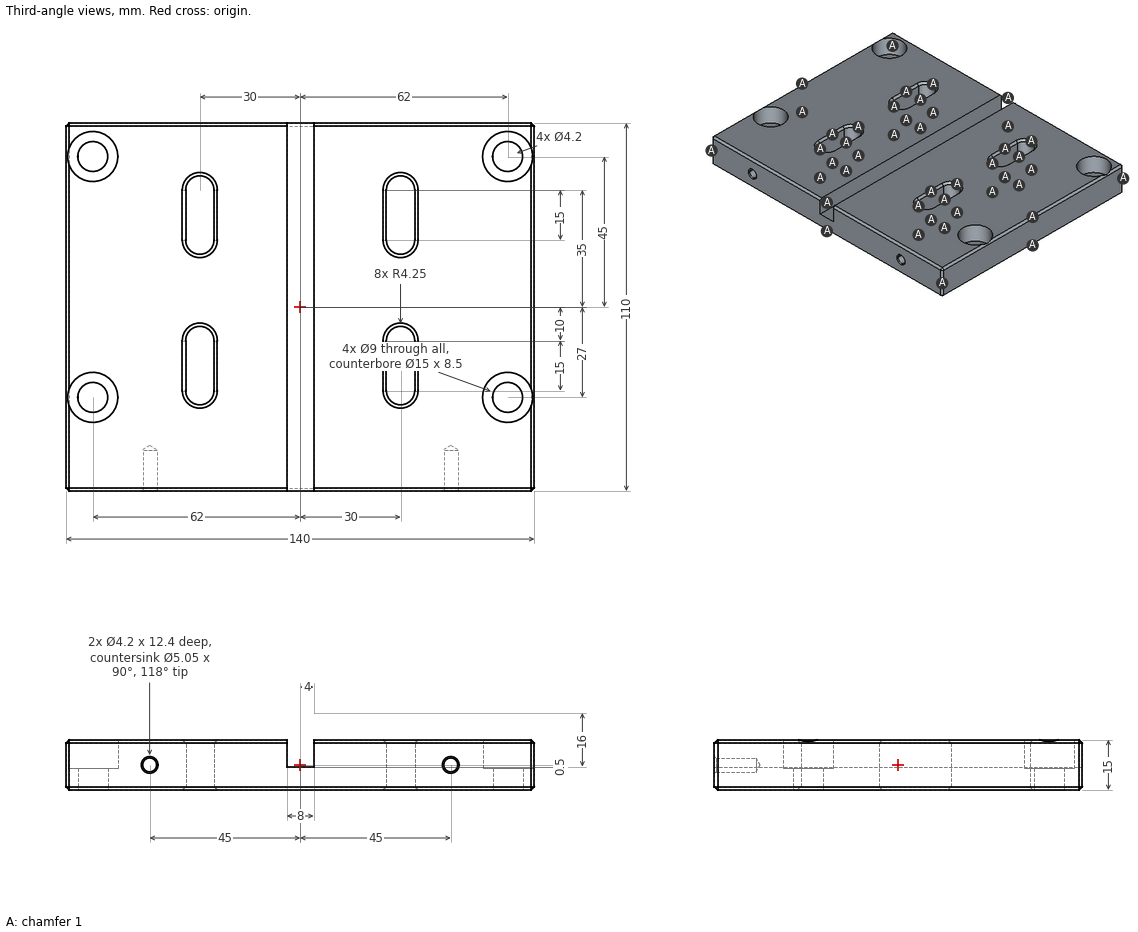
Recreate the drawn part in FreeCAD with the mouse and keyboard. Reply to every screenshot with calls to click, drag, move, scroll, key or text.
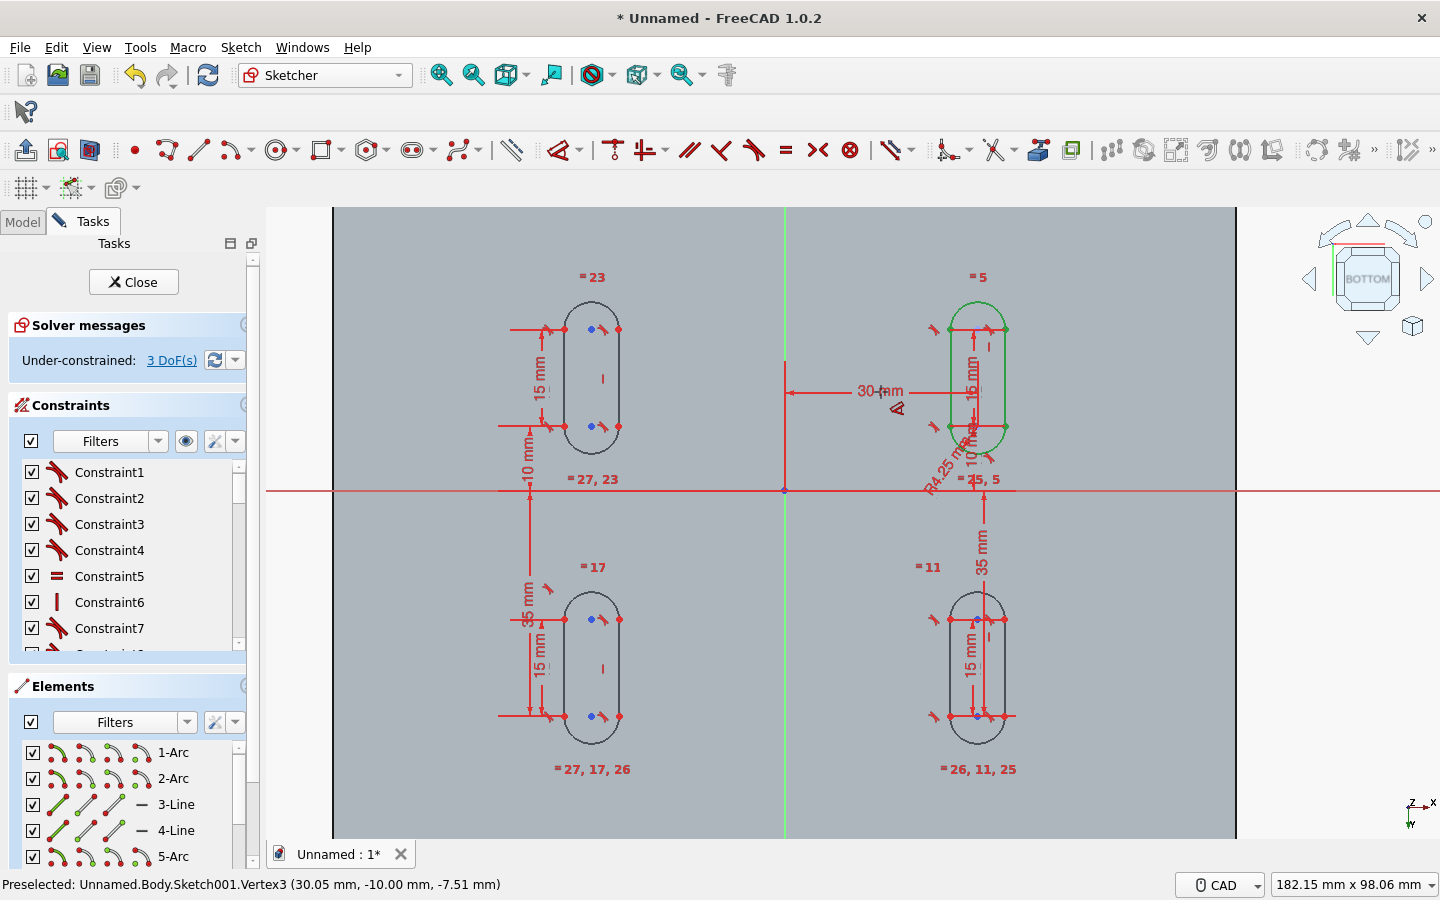
click(977, 716)
click(881, 750)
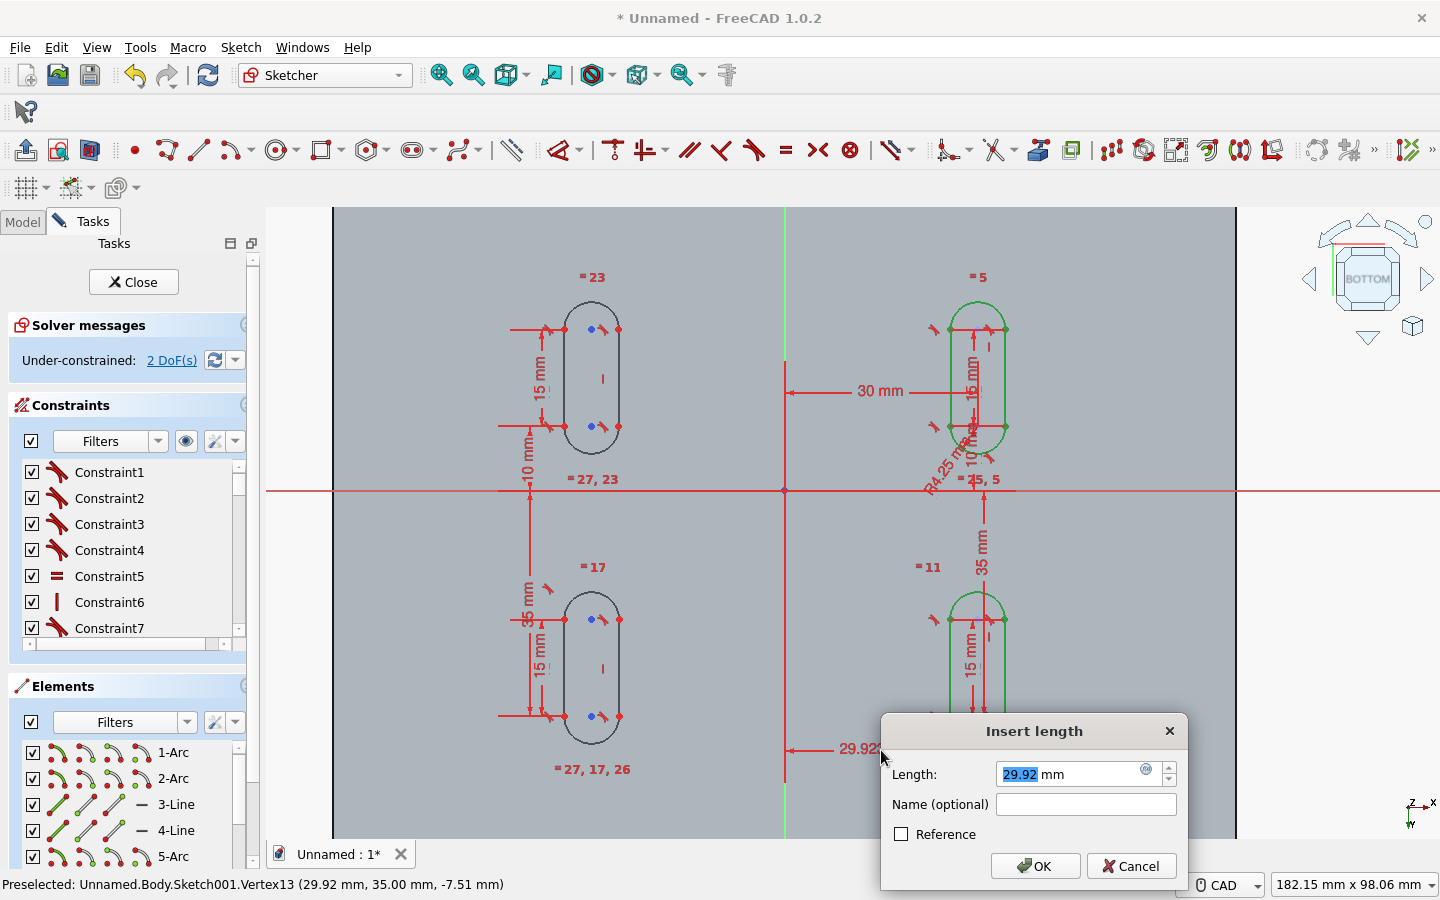
text(30)
key(Return)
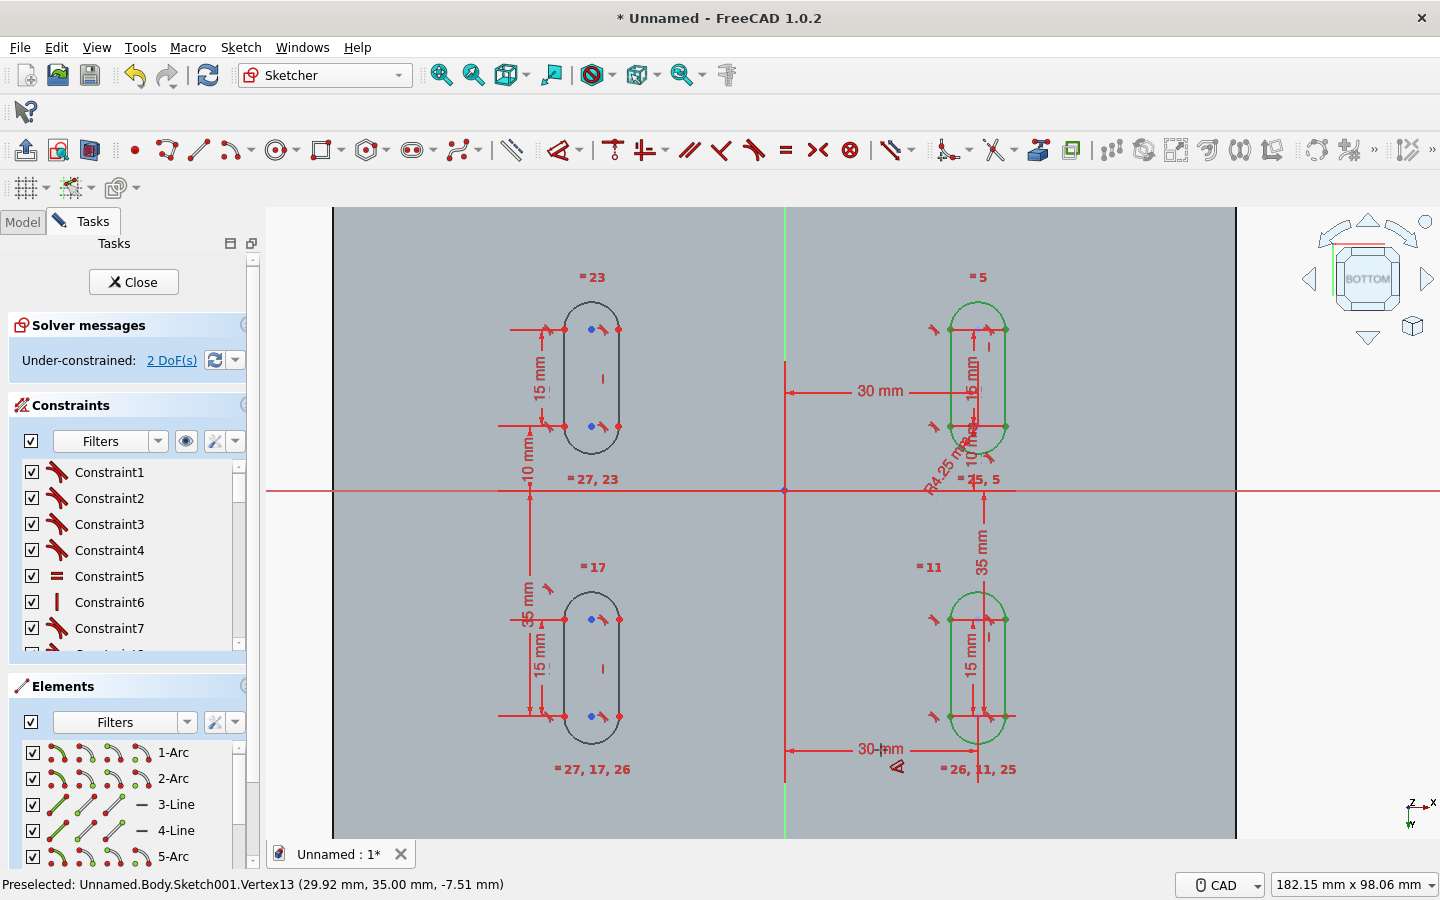
click(592, 716)
click(688, 750)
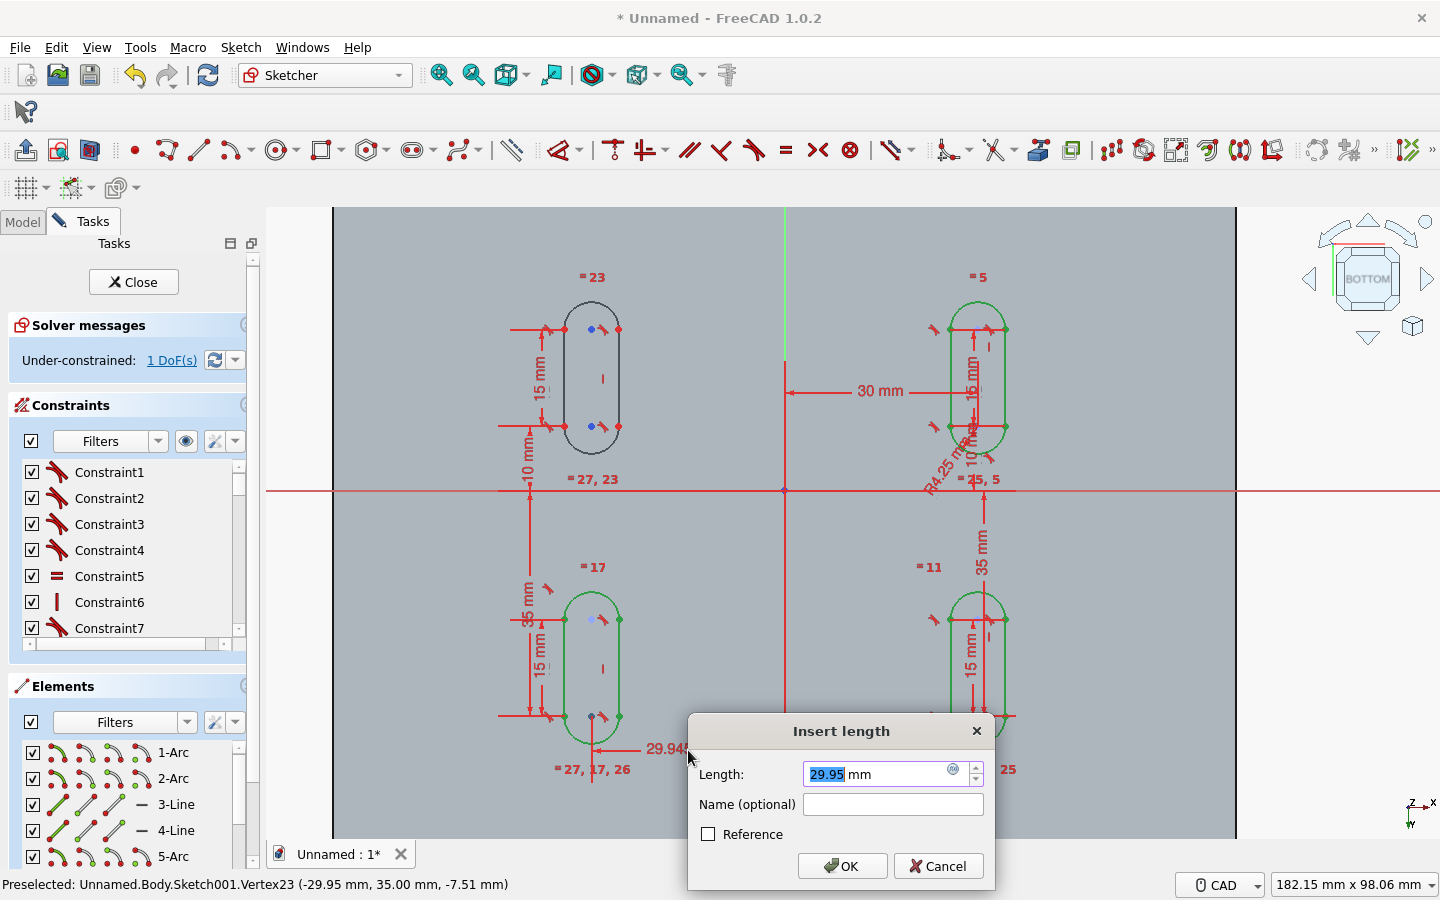
text(30)
key(Return)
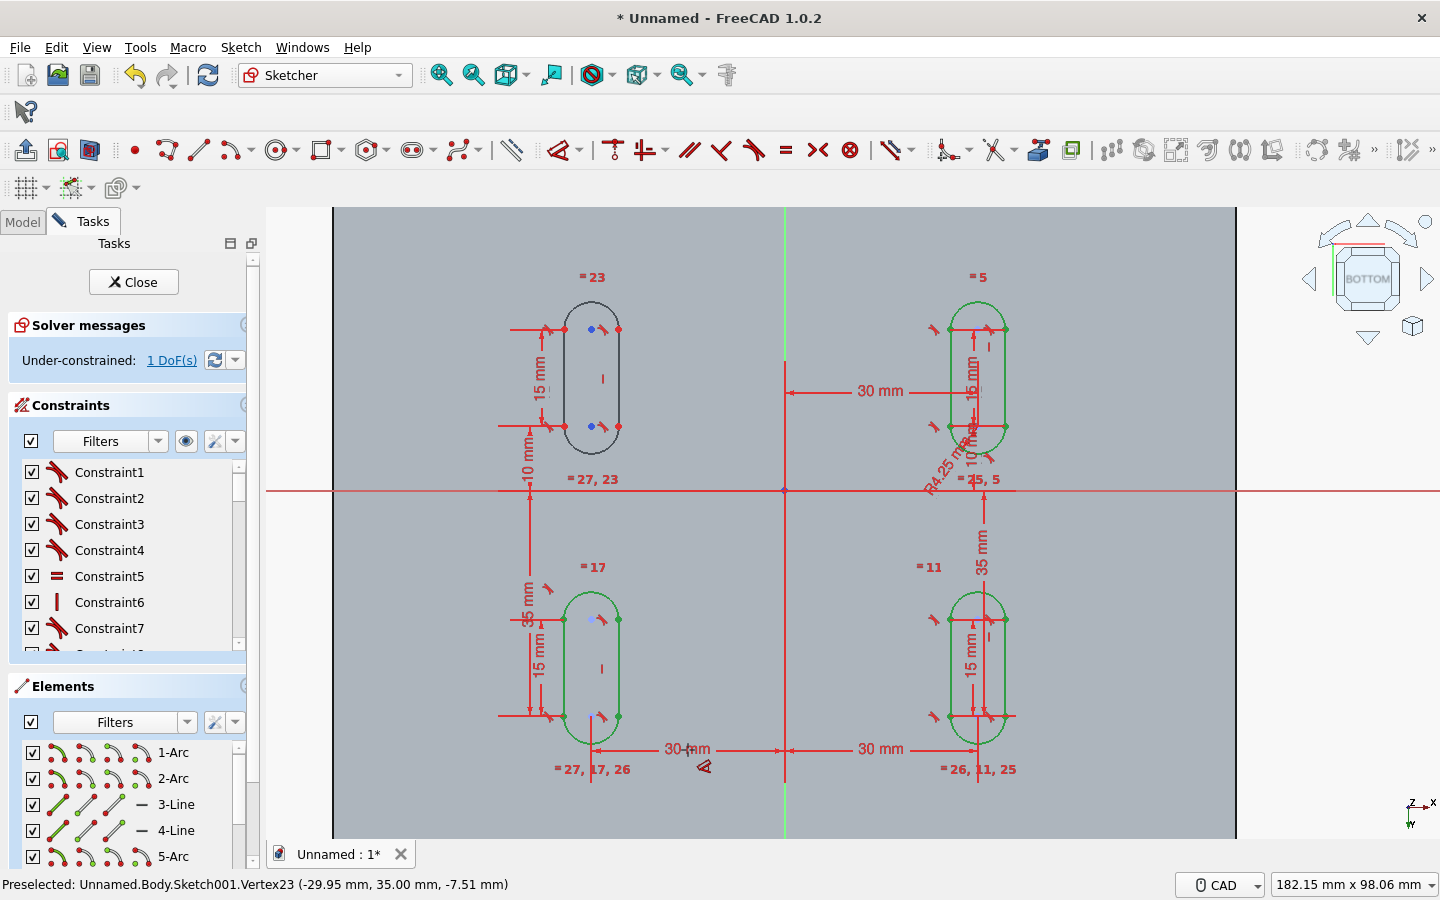
click(592, 426)
click(688, 392)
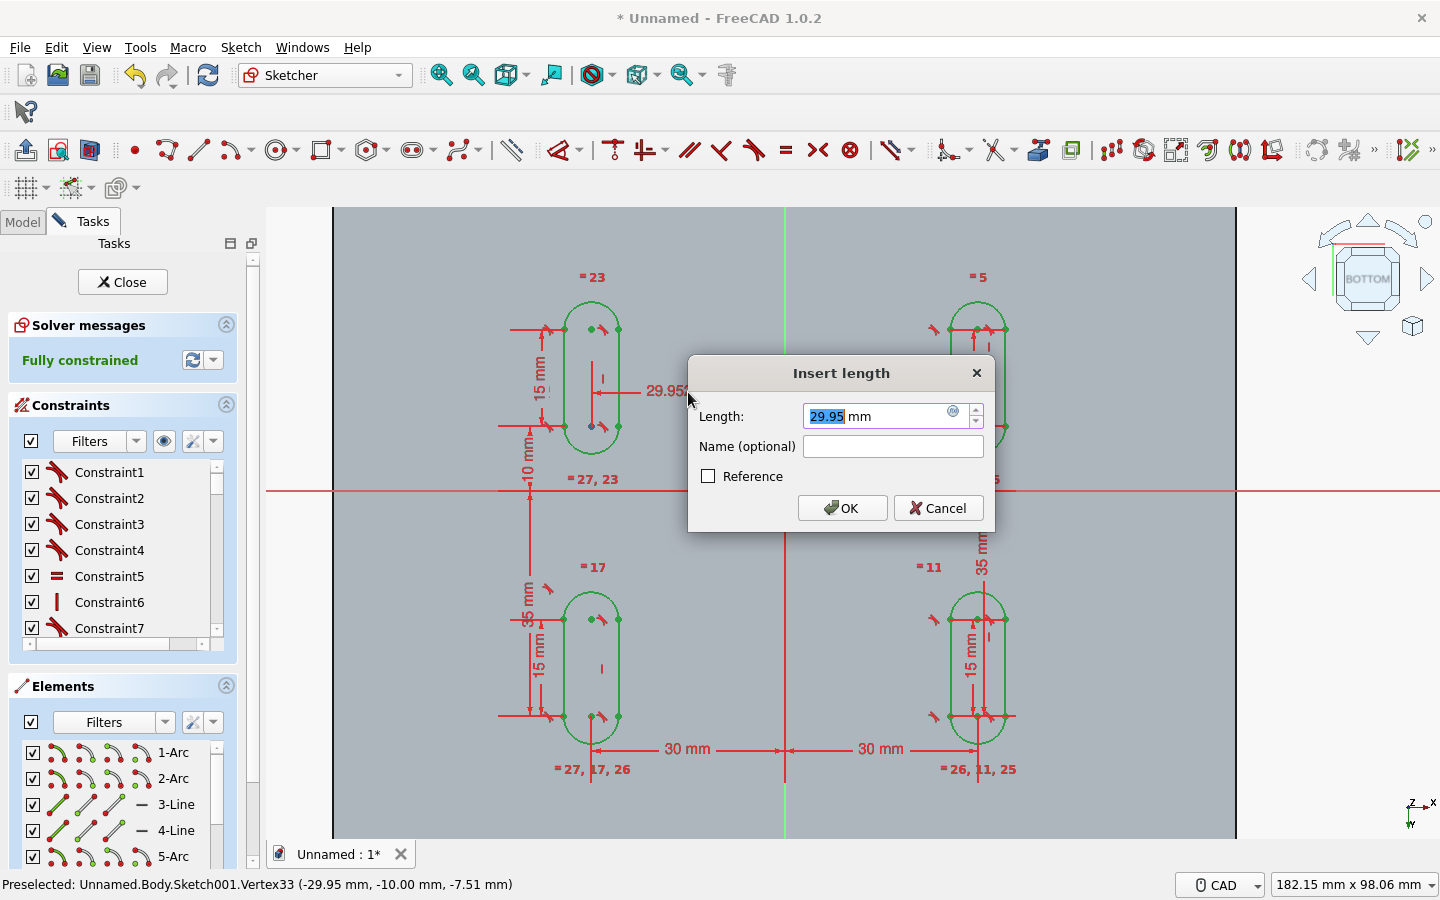
text(30)
key(Return)
key(Escape)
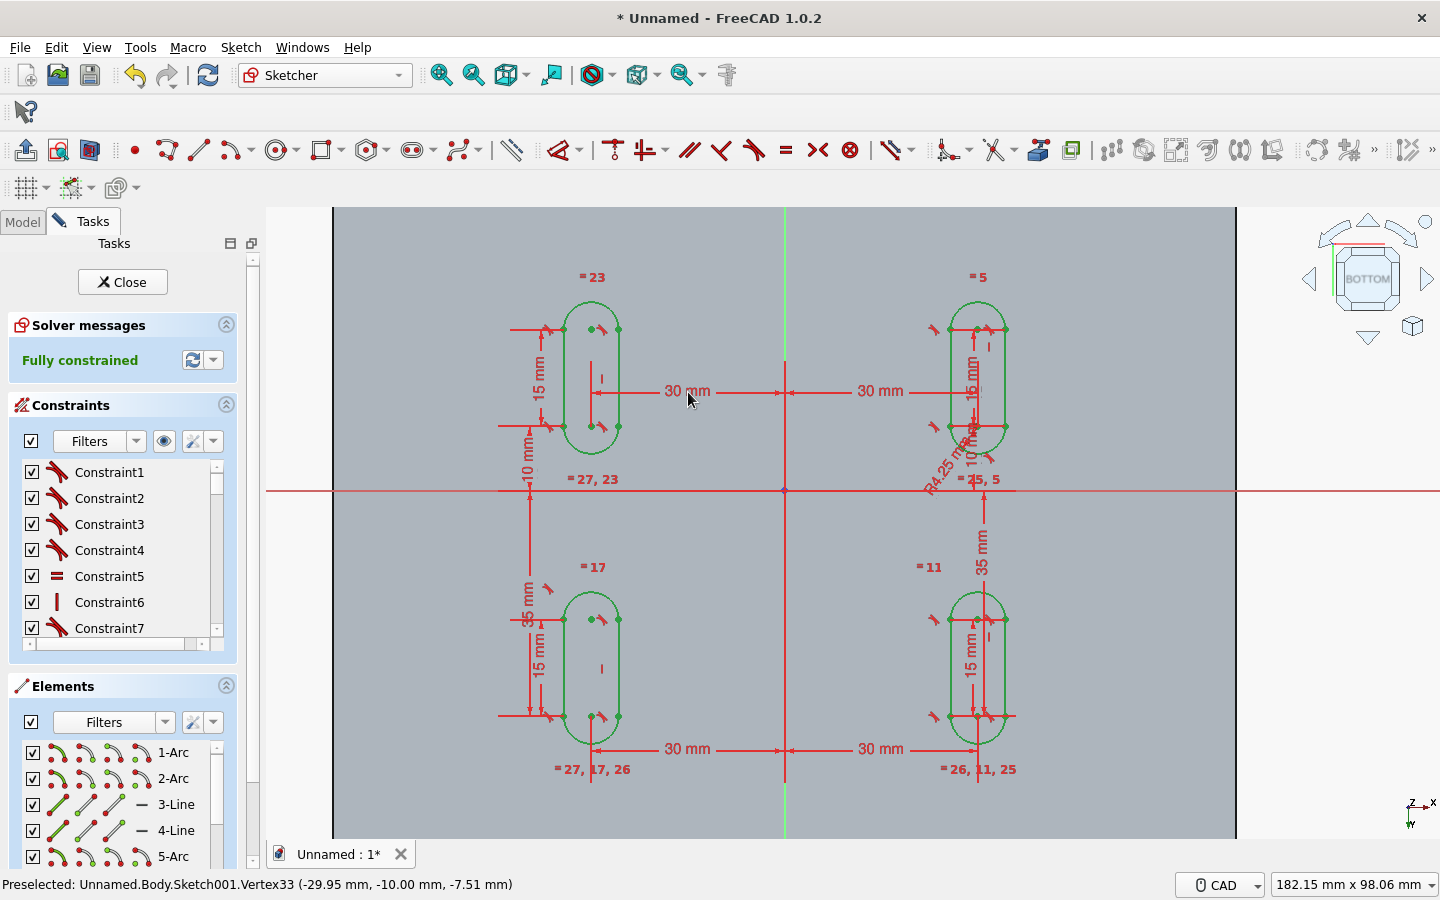
click(123, 282)